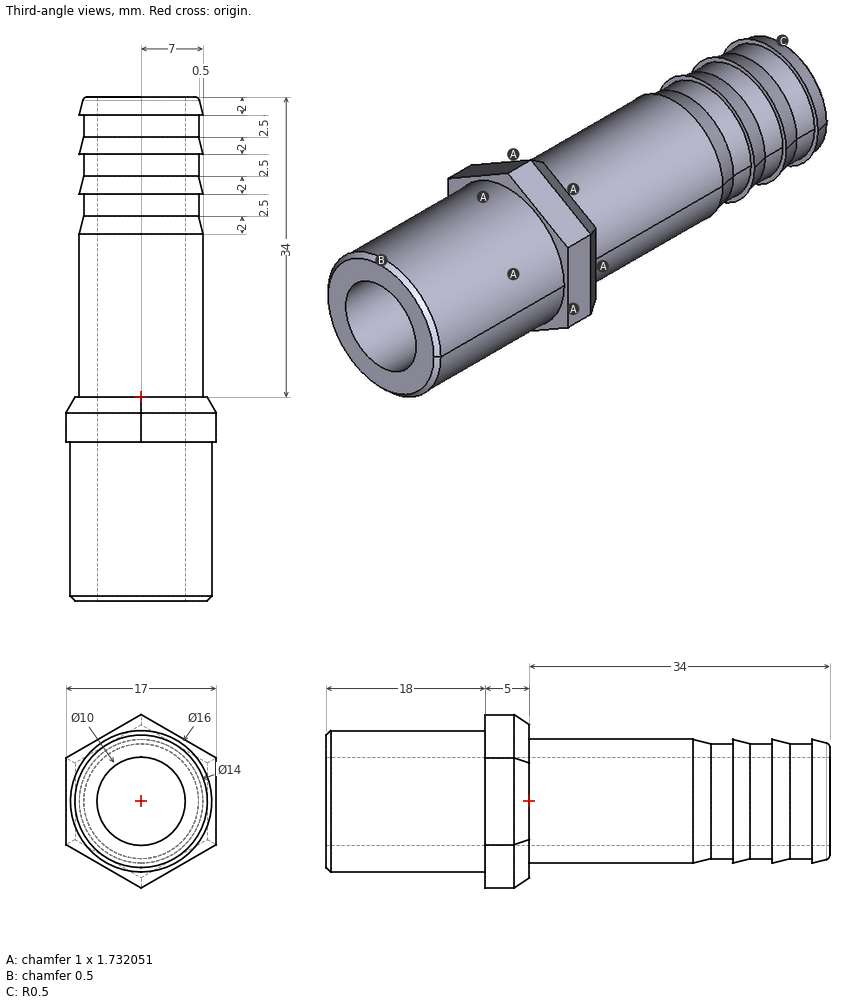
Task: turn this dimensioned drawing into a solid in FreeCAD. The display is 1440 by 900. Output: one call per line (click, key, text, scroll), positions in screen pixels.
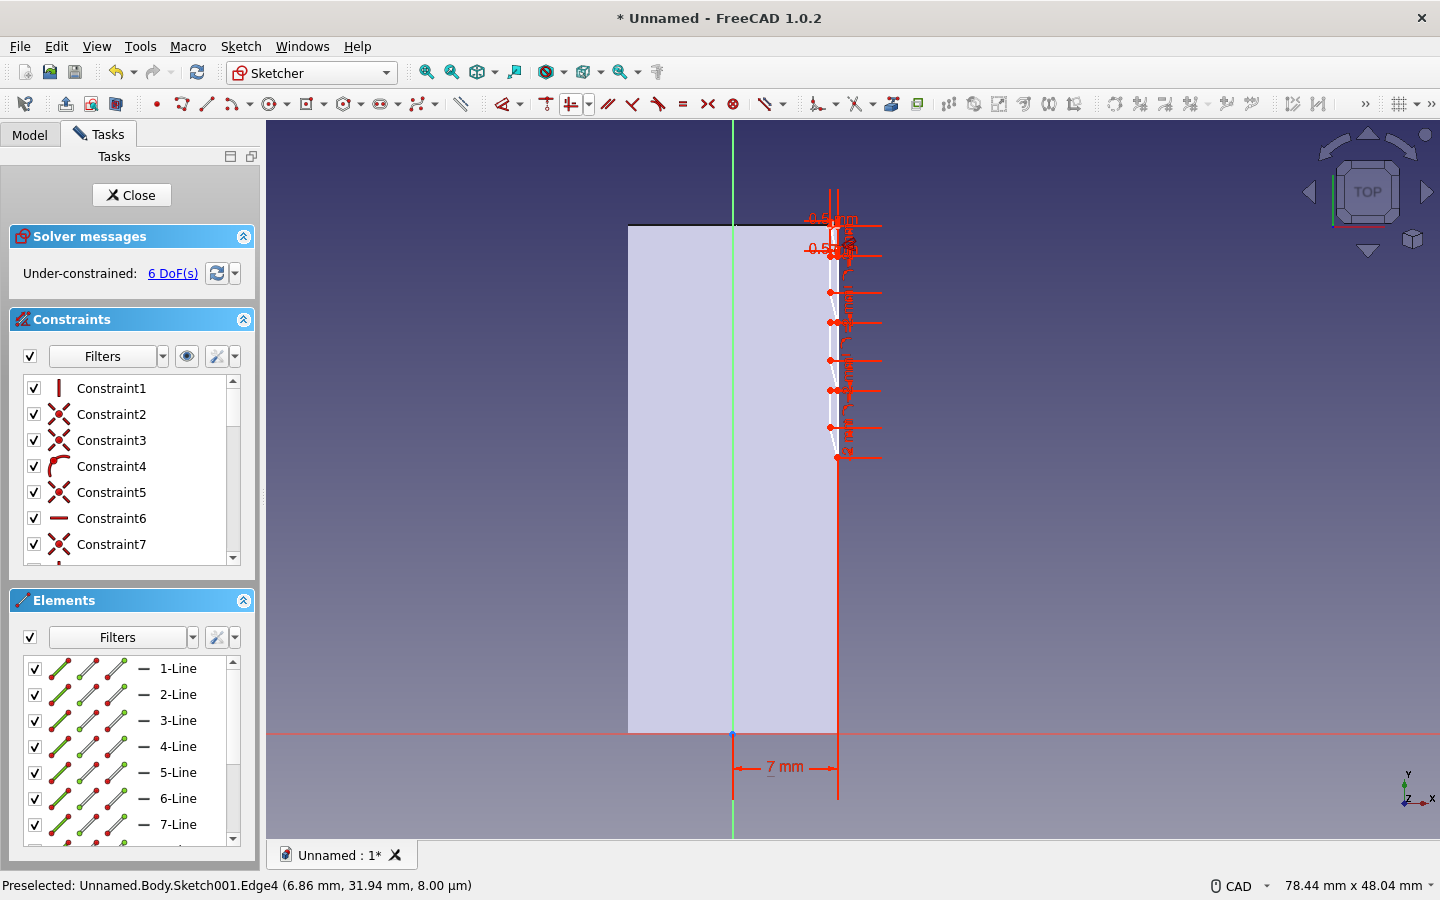
scroll(830, 267, up, 4)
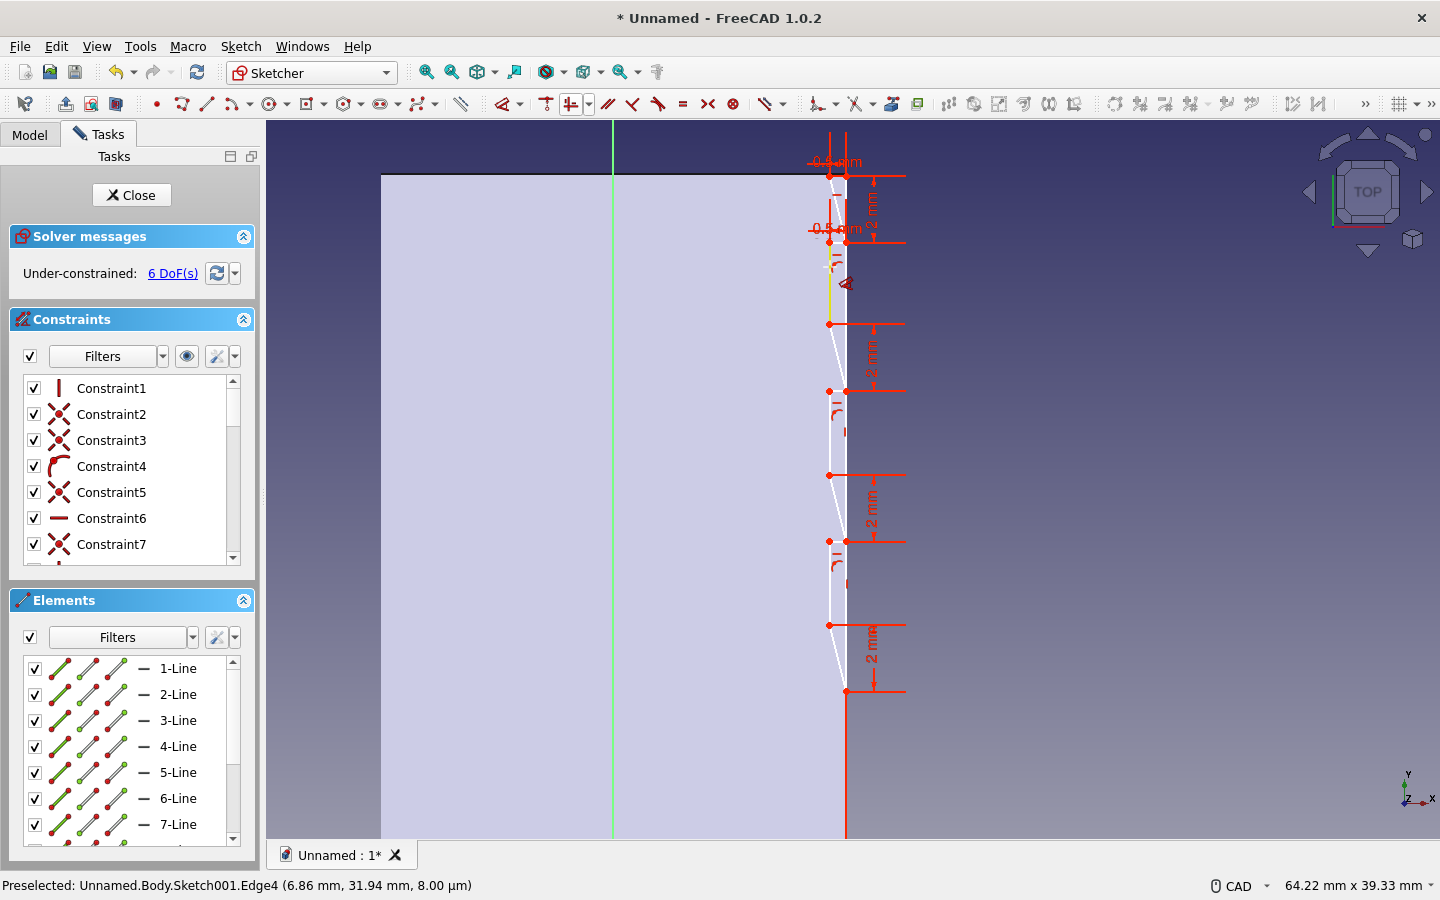
click(830, 267)
click(864, 284)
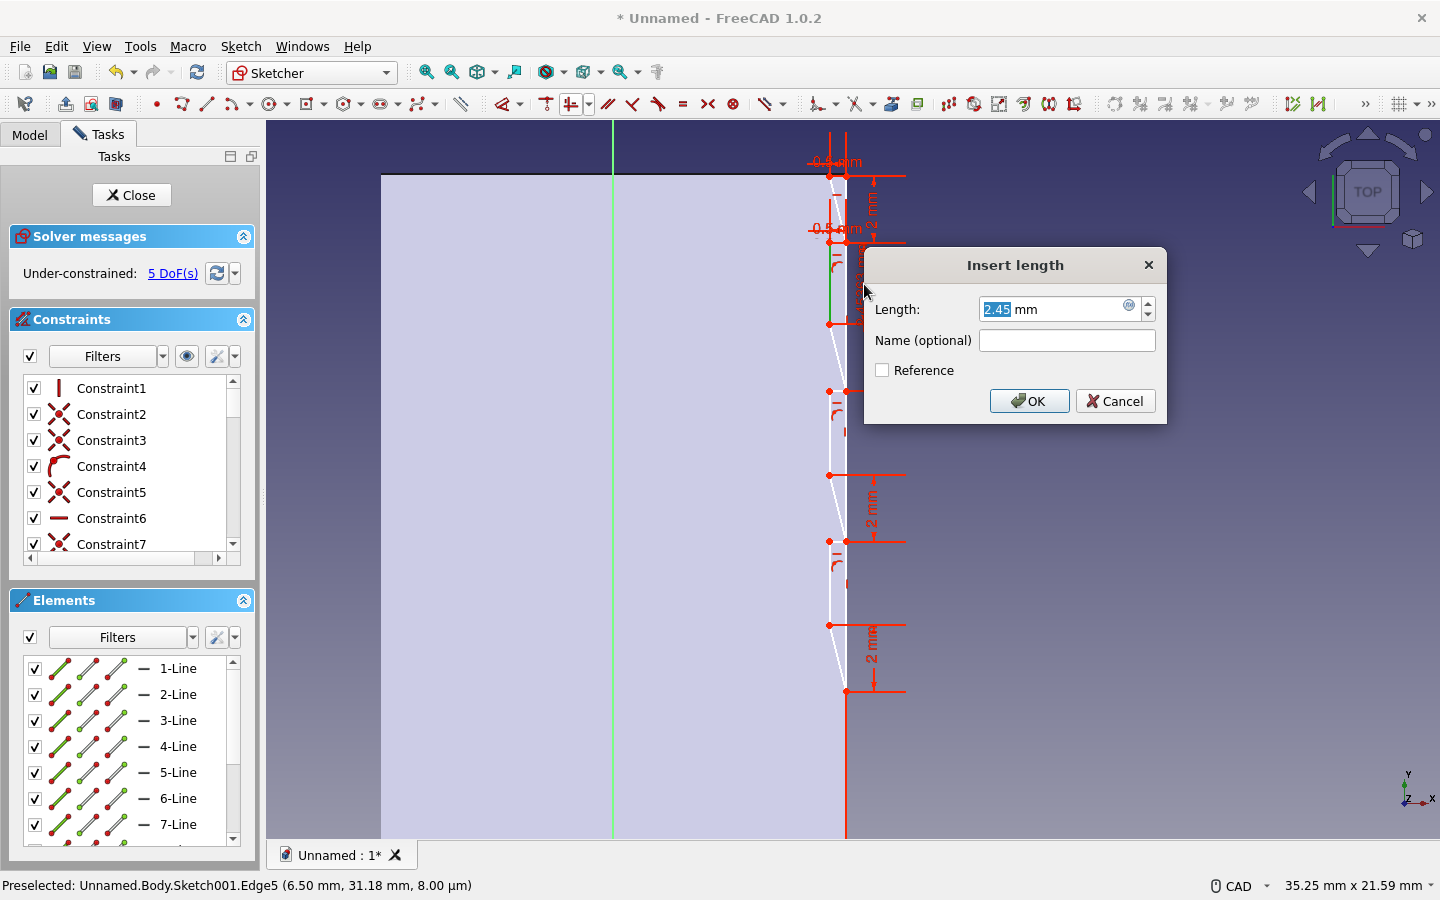
text(2.5)
key(Return)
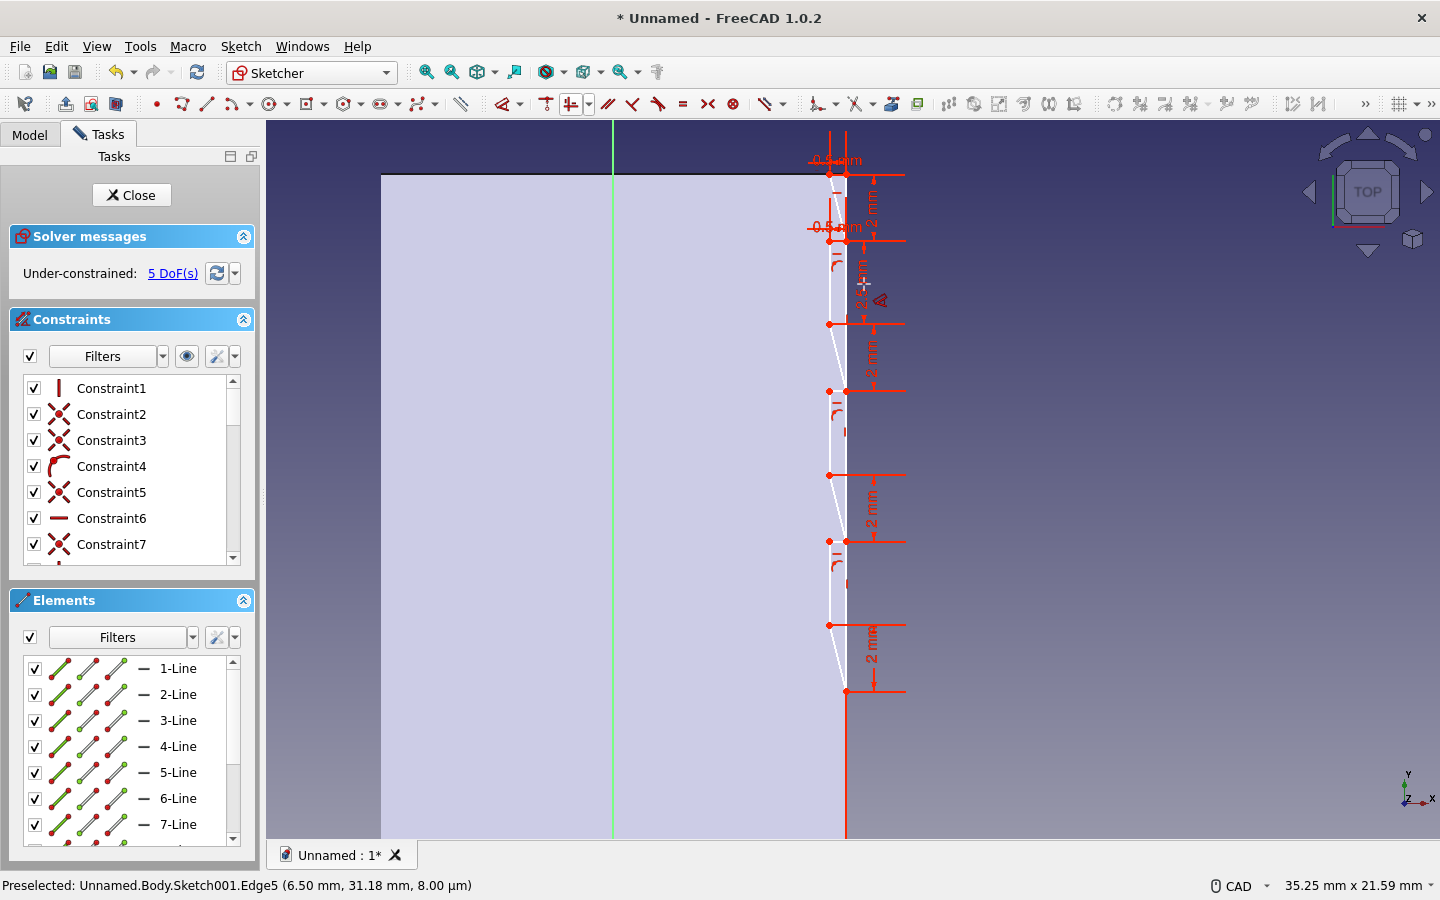
scroll(838, 391, up, 5)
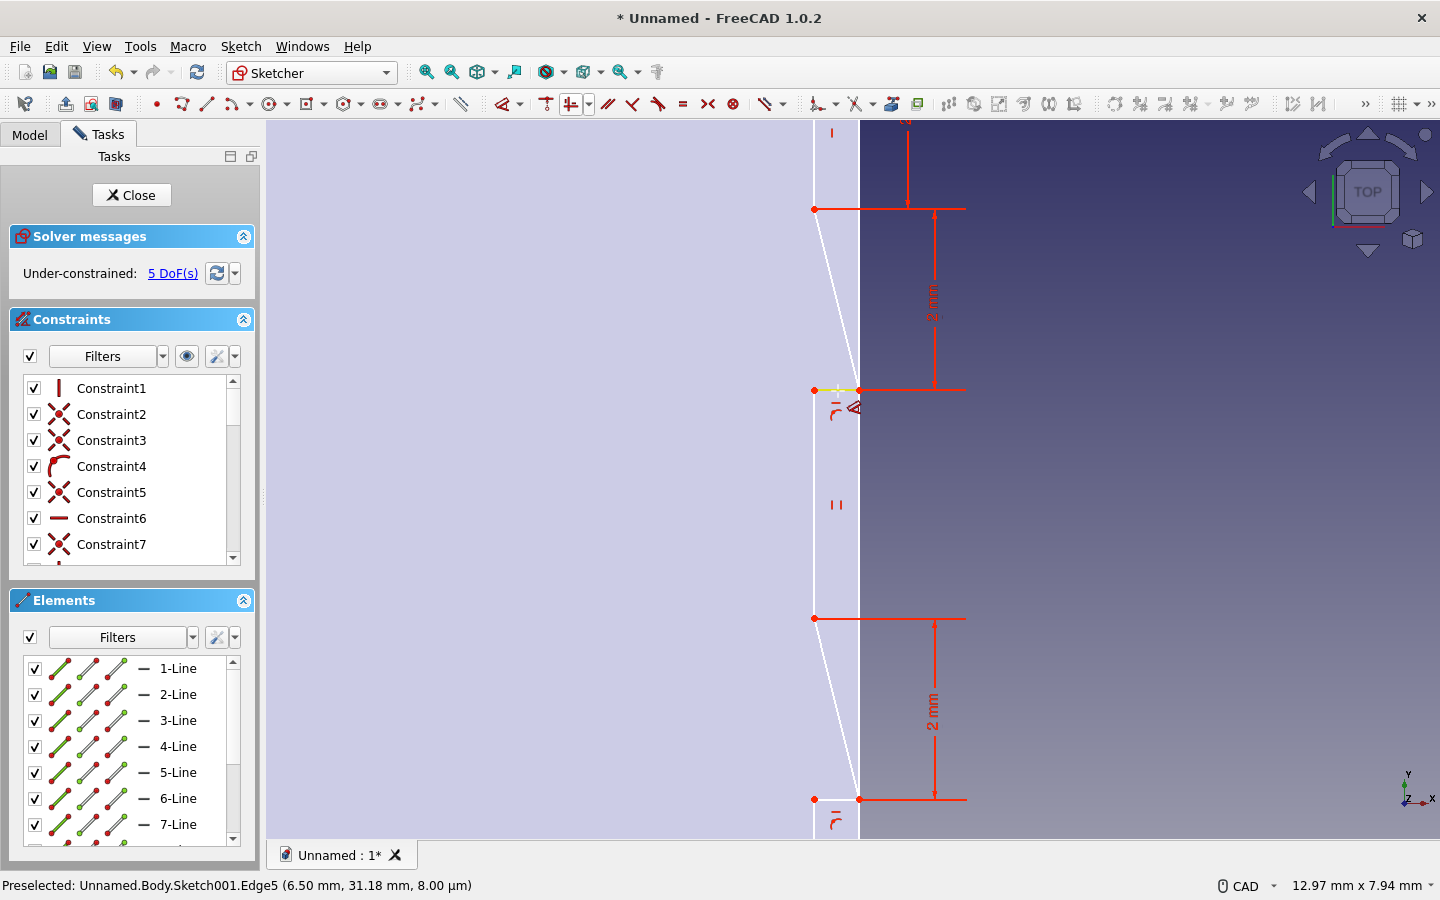
click(837, 390)
click(837, 356)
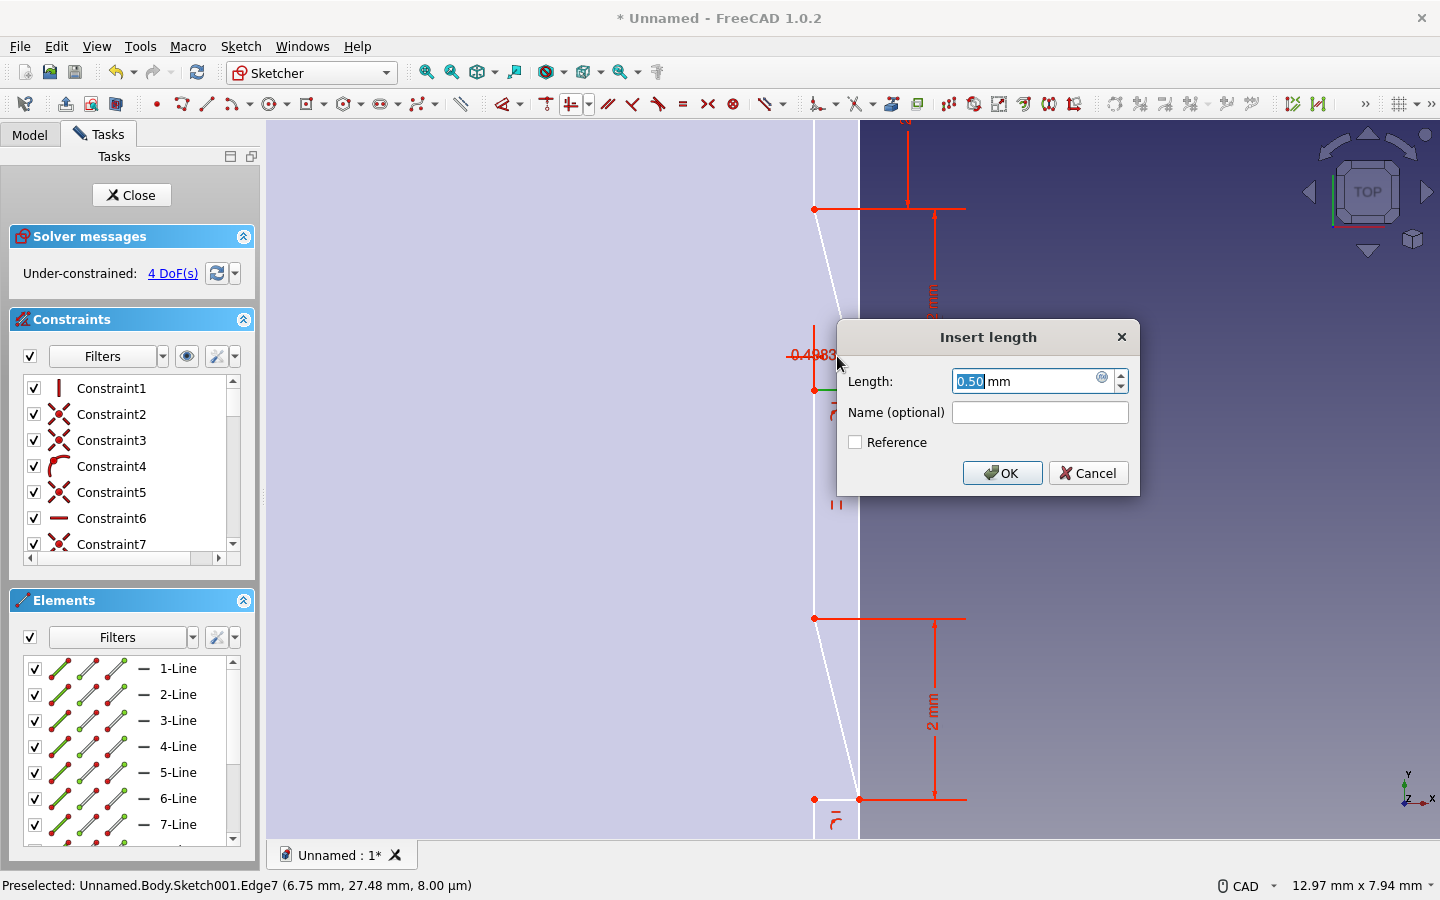
text(0.5)
key(Return)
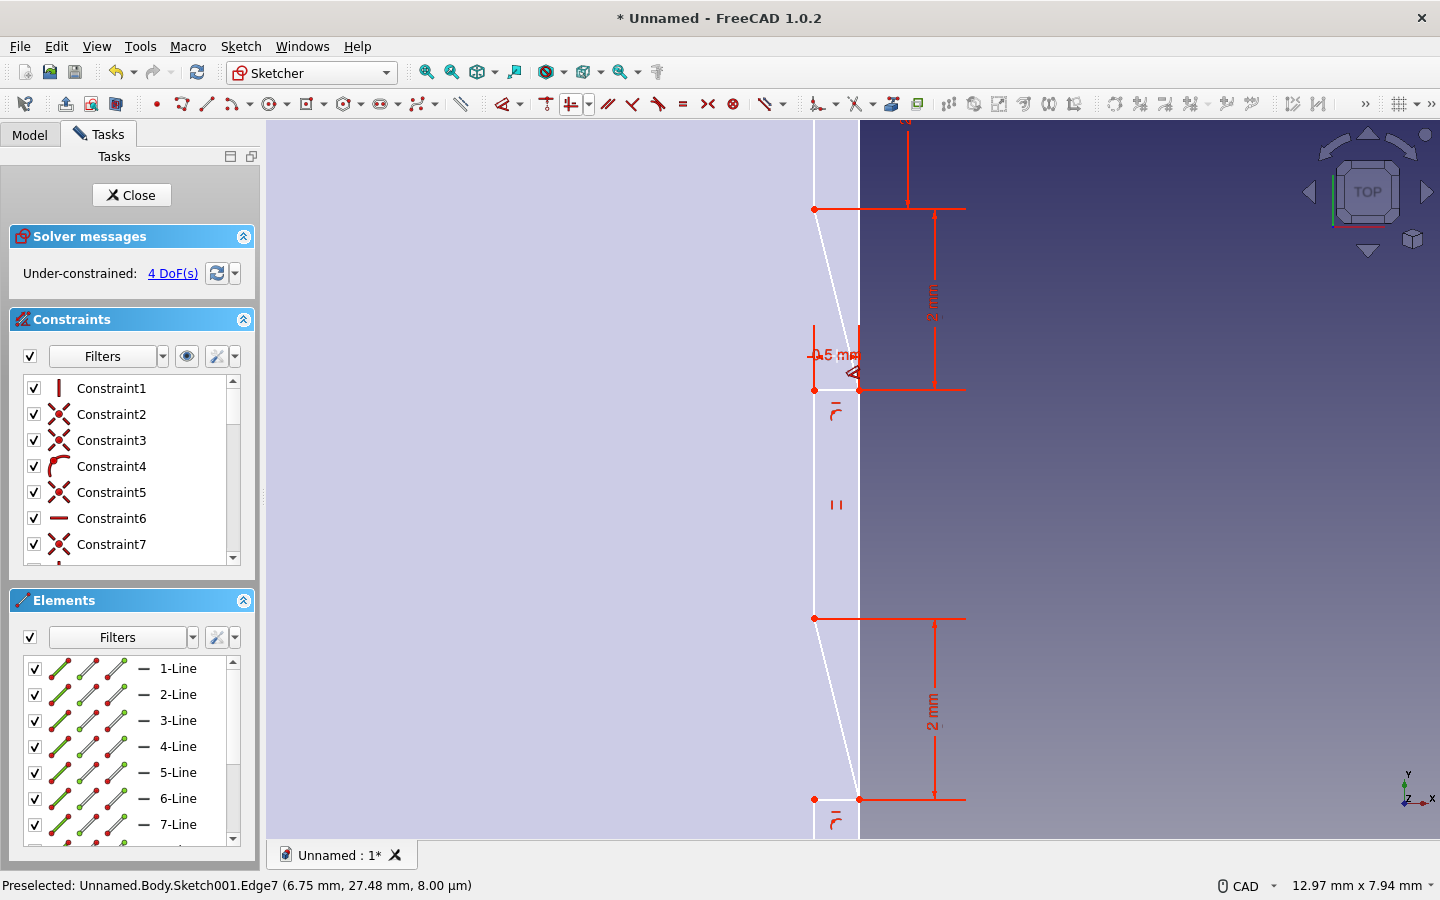
scroll(832, 309, down, 9)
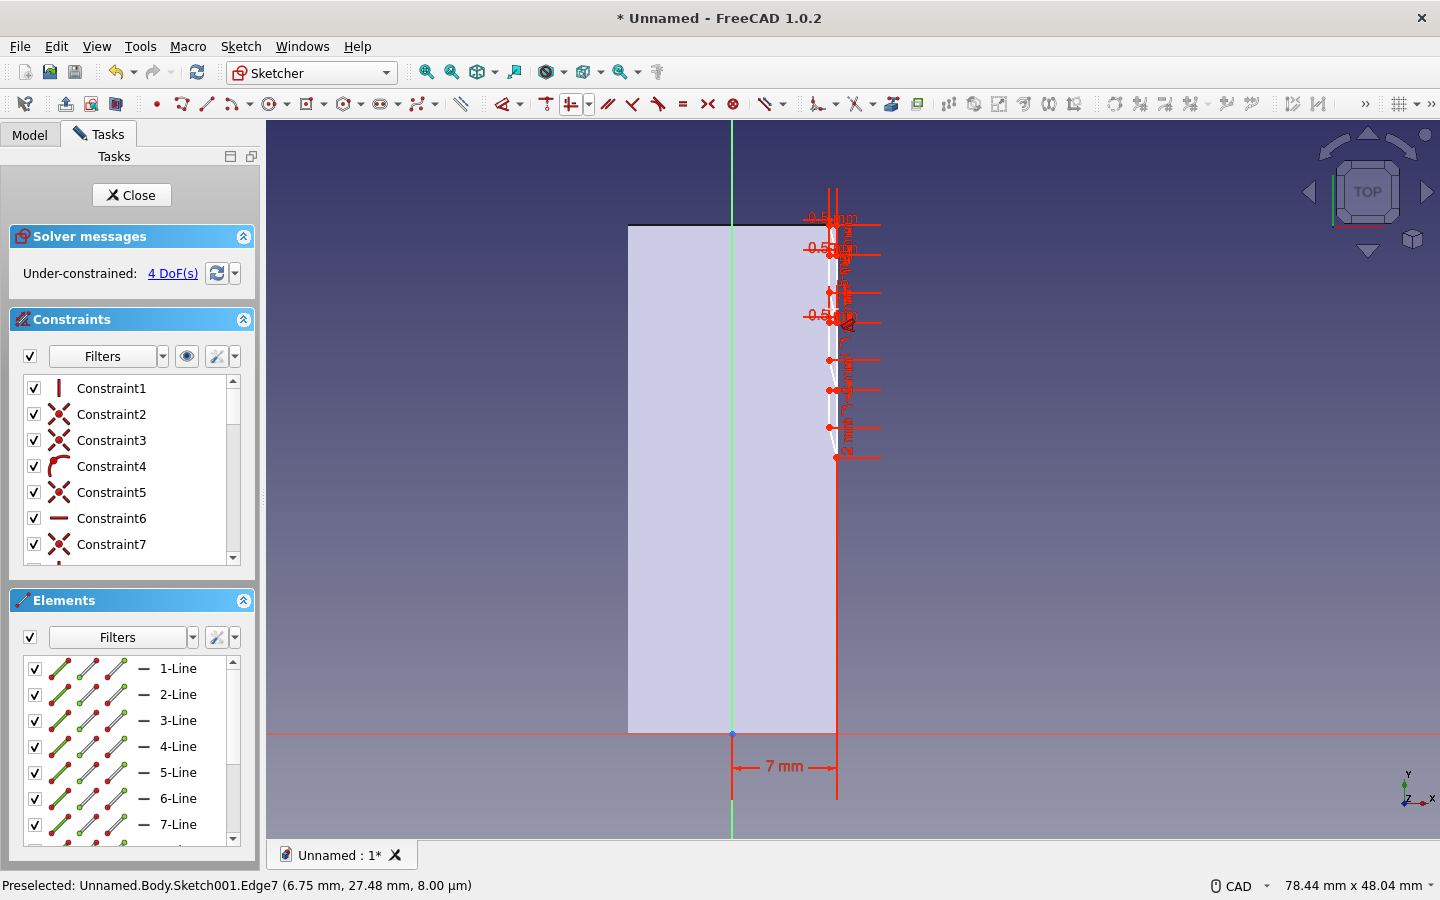
scroll(829, 334, up, 4)